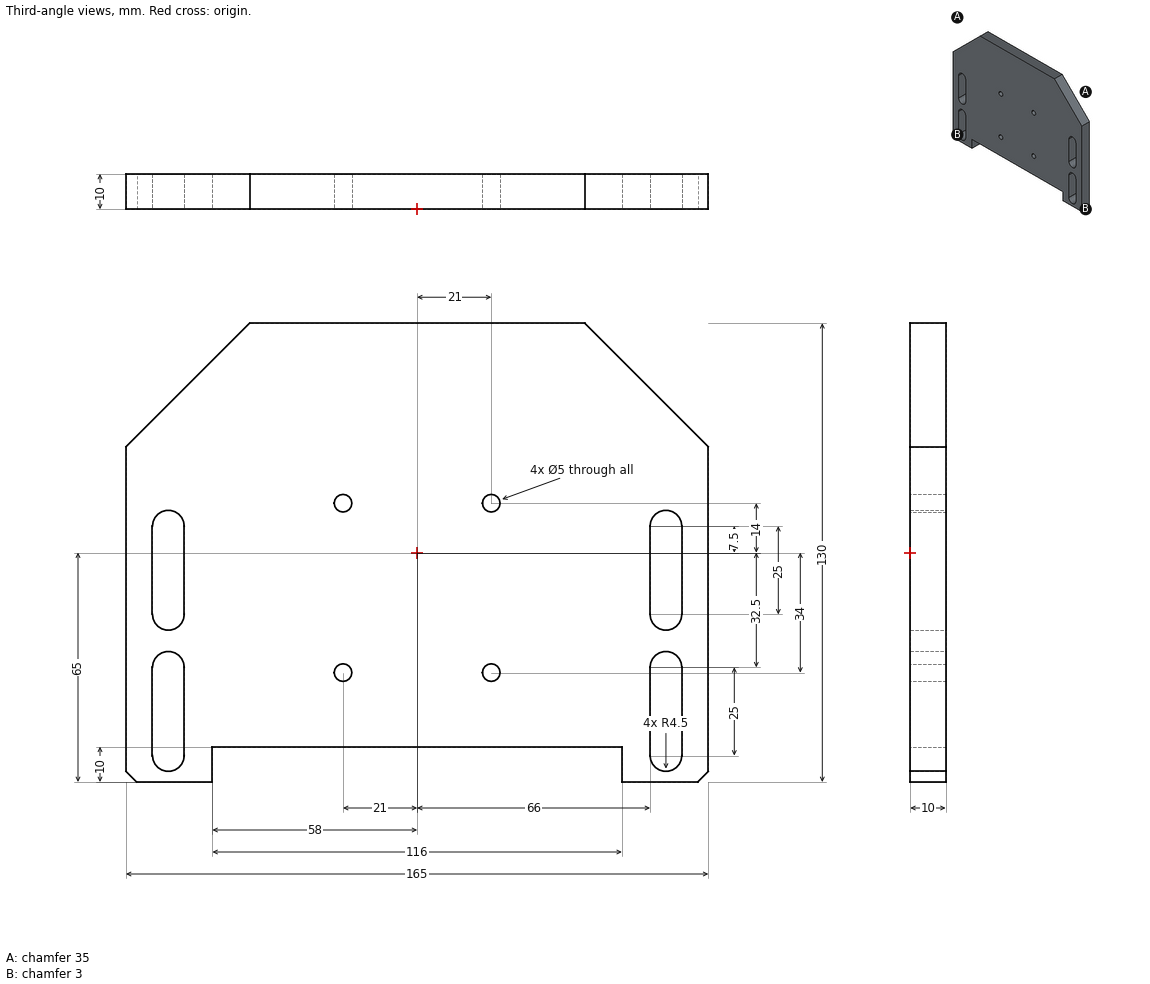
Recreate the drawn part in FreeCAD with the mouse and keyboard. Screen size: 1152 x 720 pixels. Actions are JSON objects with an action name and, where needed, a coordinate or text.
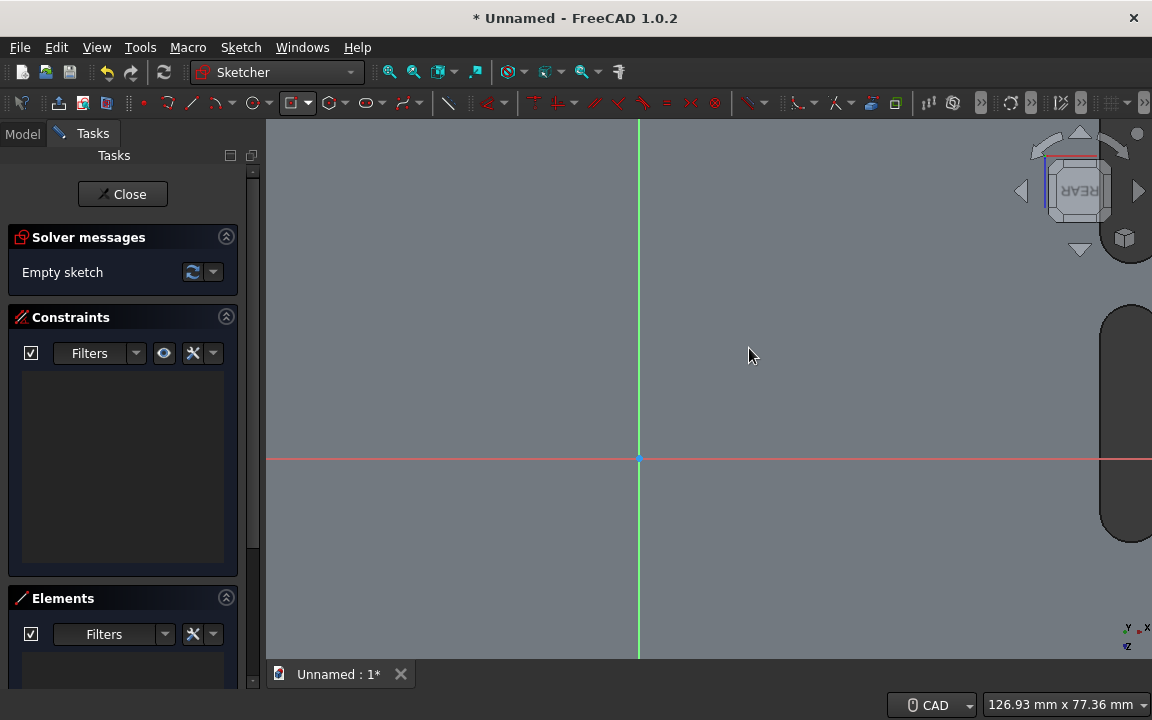
{"action": "left_click", "coordinate": [254, 104]}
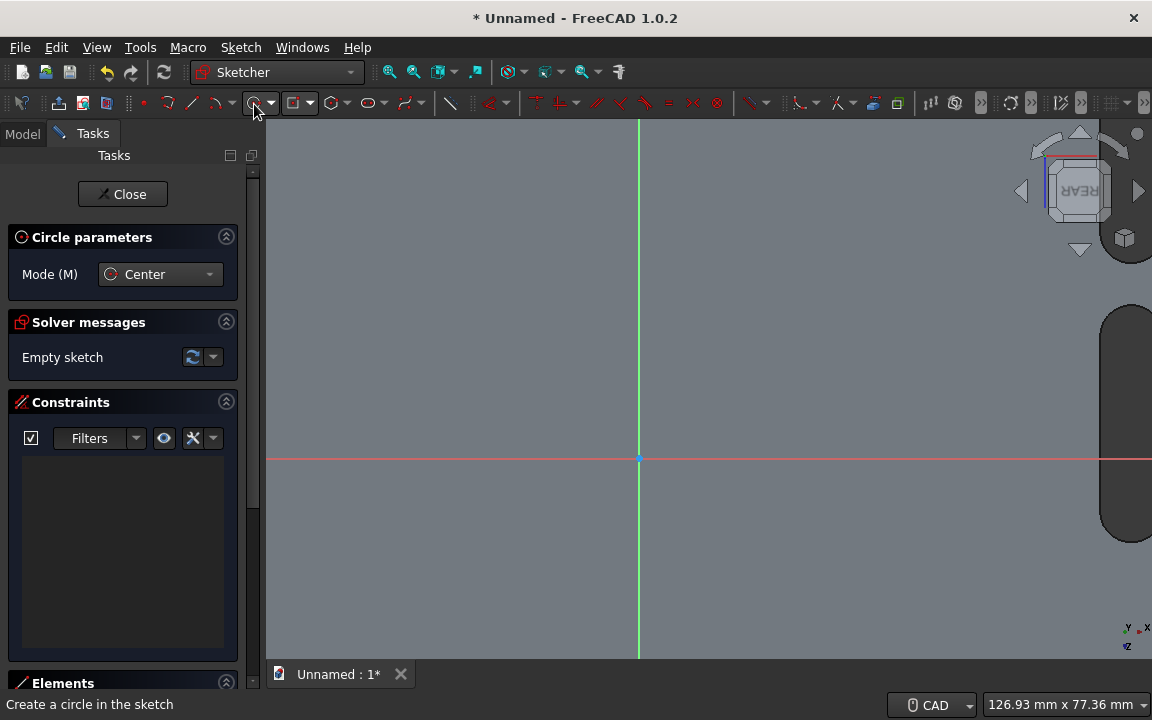
{"action": "scroll", "coordinate": [786, 556], "scroll_direction": "up", "scroll_amount": 2}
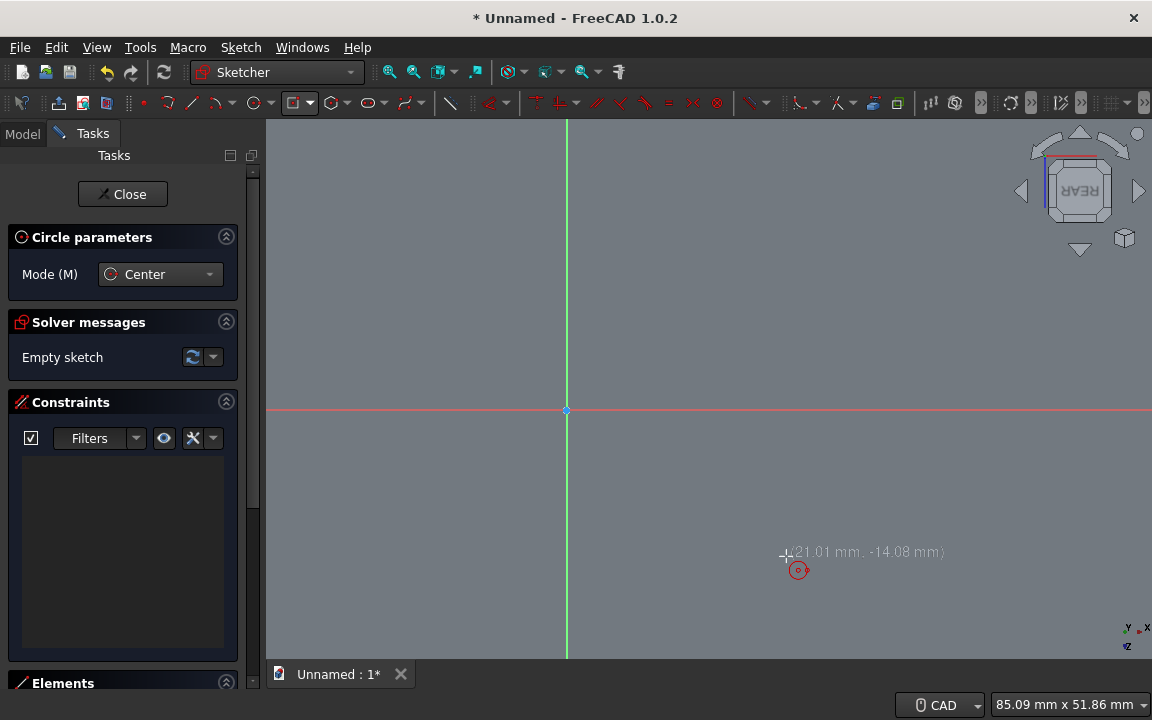
{"action": "left_click", "coordinate": [786, 556]}
{"action": "left_click", "coordinate": [804, 538]}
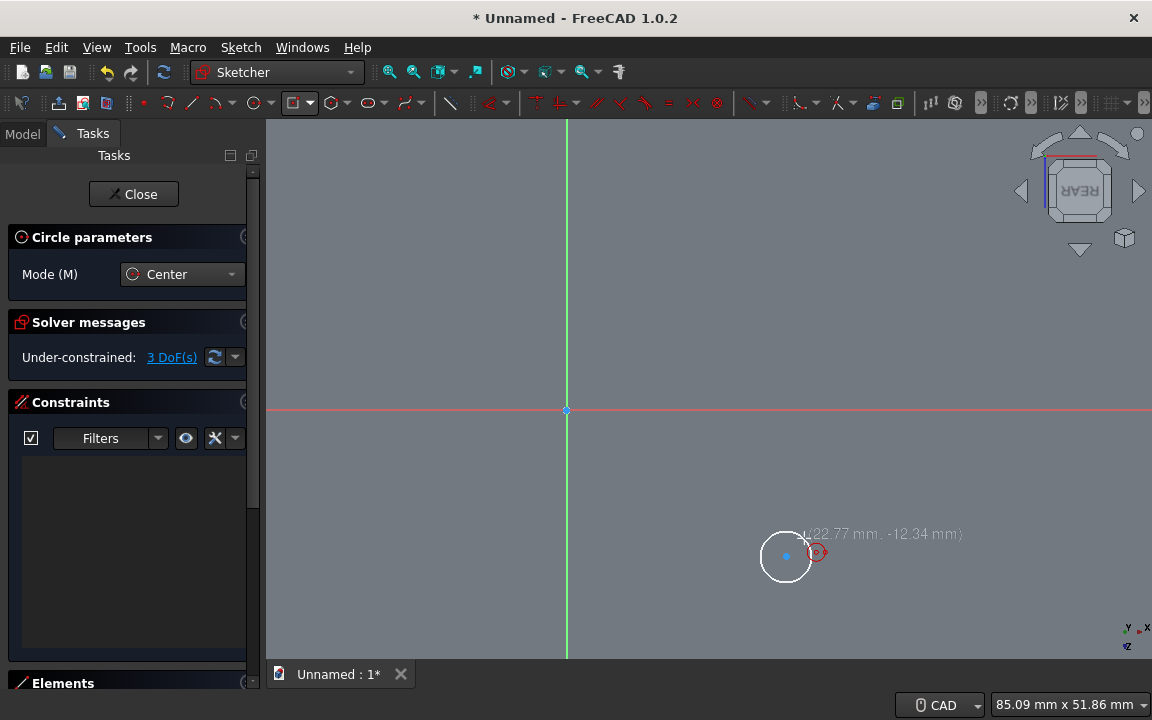
{"action": "scroll", "coordinate": [790, 557], "scroll_direction": "down", "scroll_amount": 2}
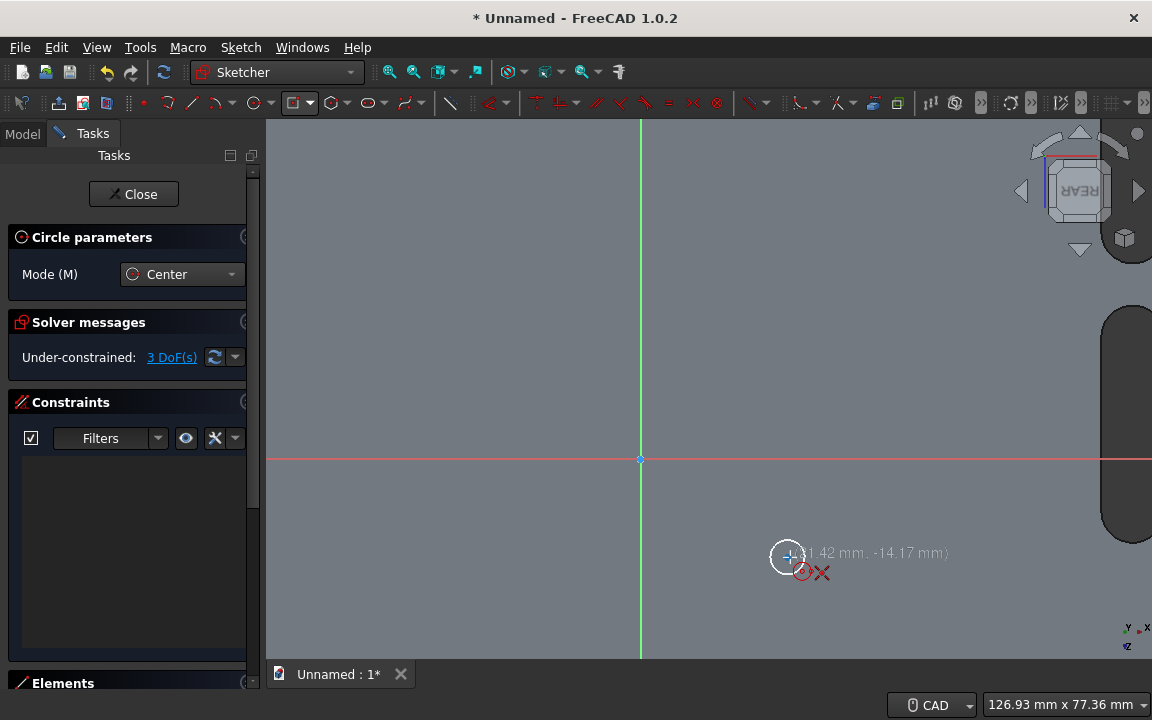
{"action": "scroll", "coordinate": [787, 222], "scroll_direction": "up", "scroll_amount": 2}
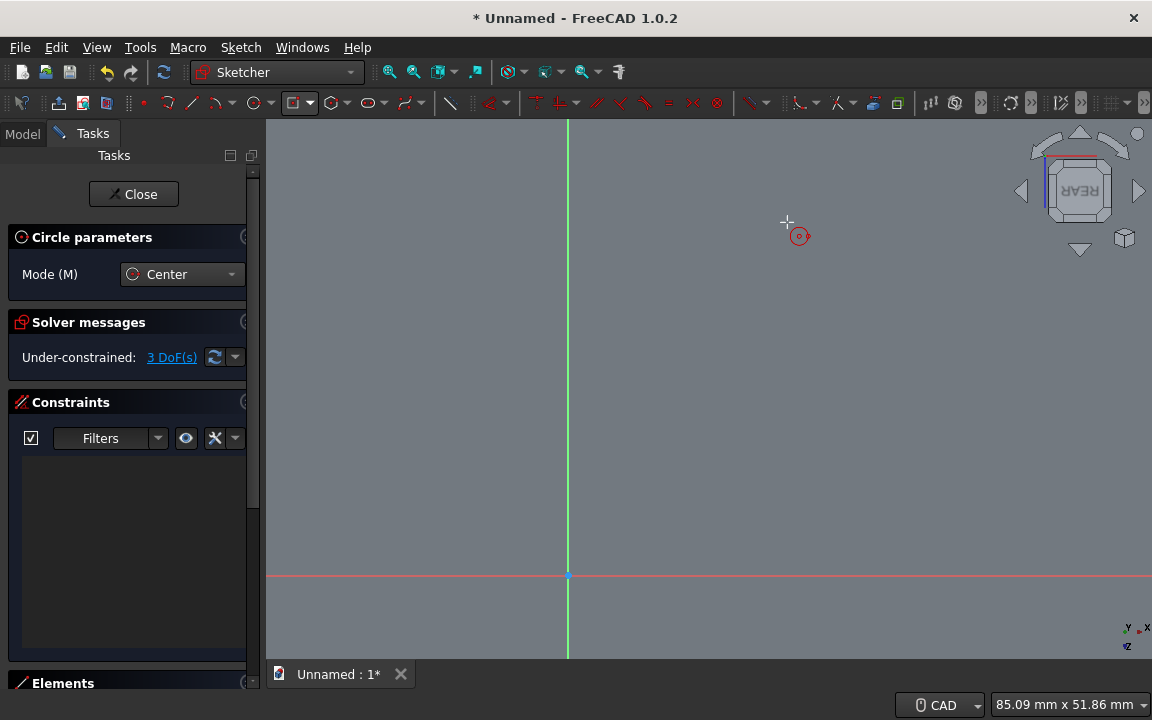
{"action": "left_click", "coordinate": [787, 222]}
{"action": "left_click", "coordinate": [805, 203]}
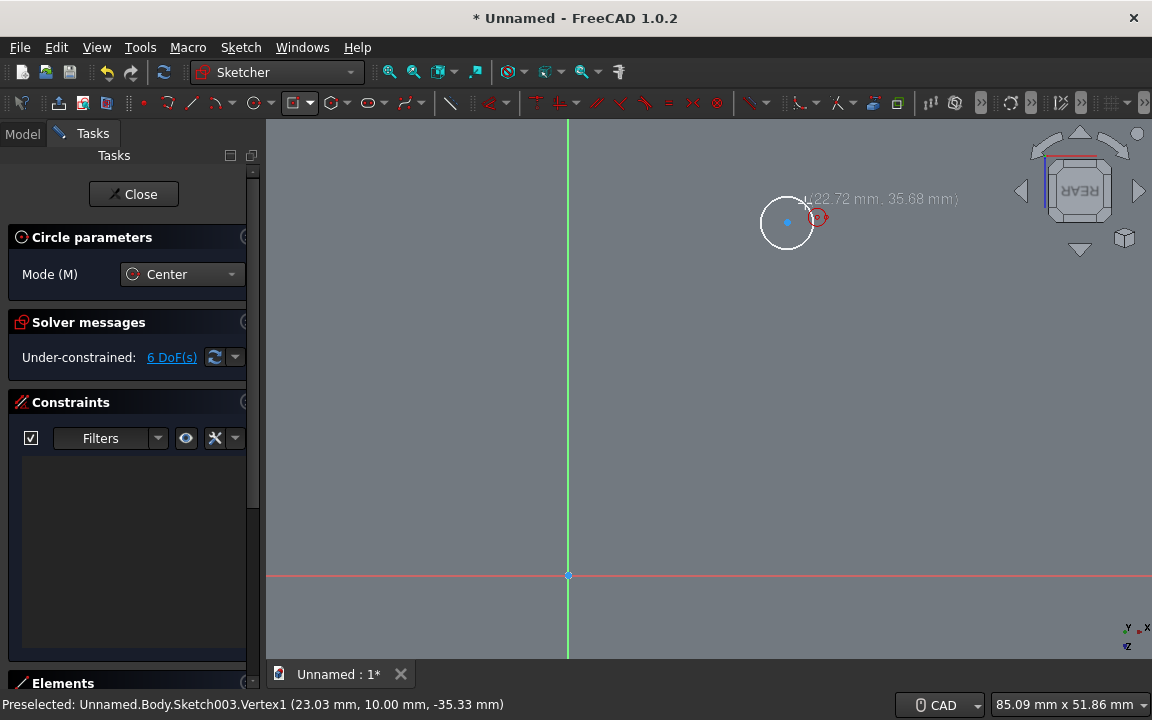
{"action": "left_click", "coordinate": [350, 222]}
{"action": "left_click", "coordinate": [368, 203]}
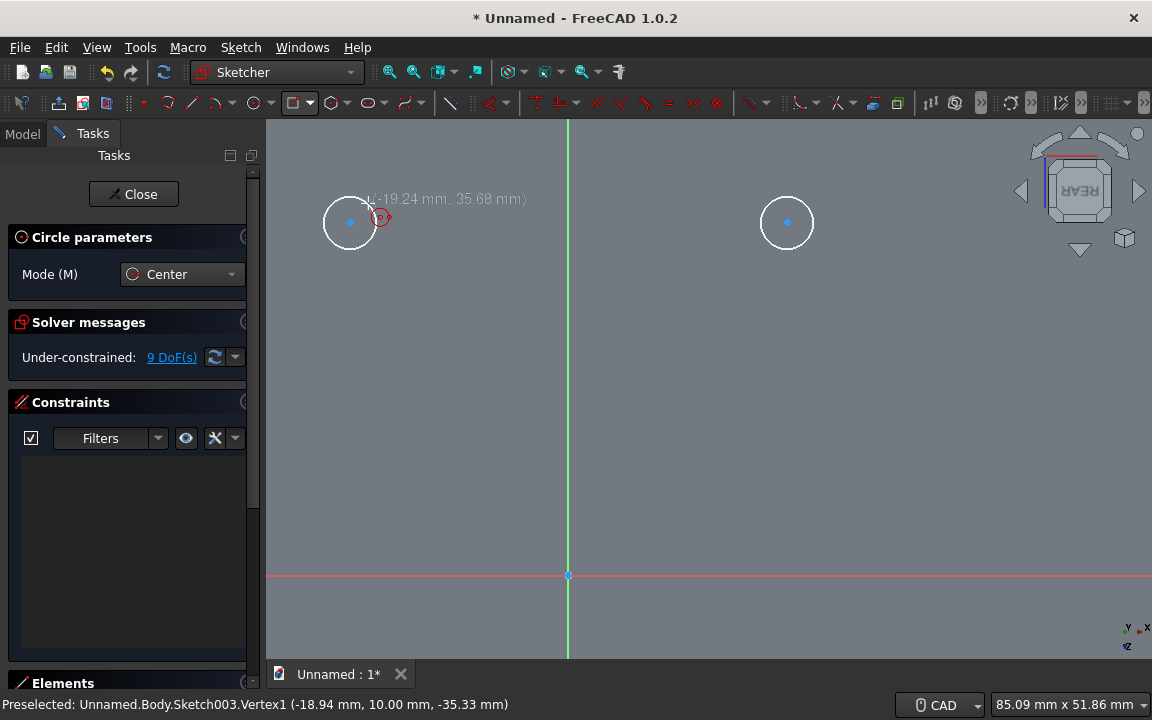
{"action": "scroll", "coordinate": [787, 221], "scroll_direction": "down", "scroll_amount": 2}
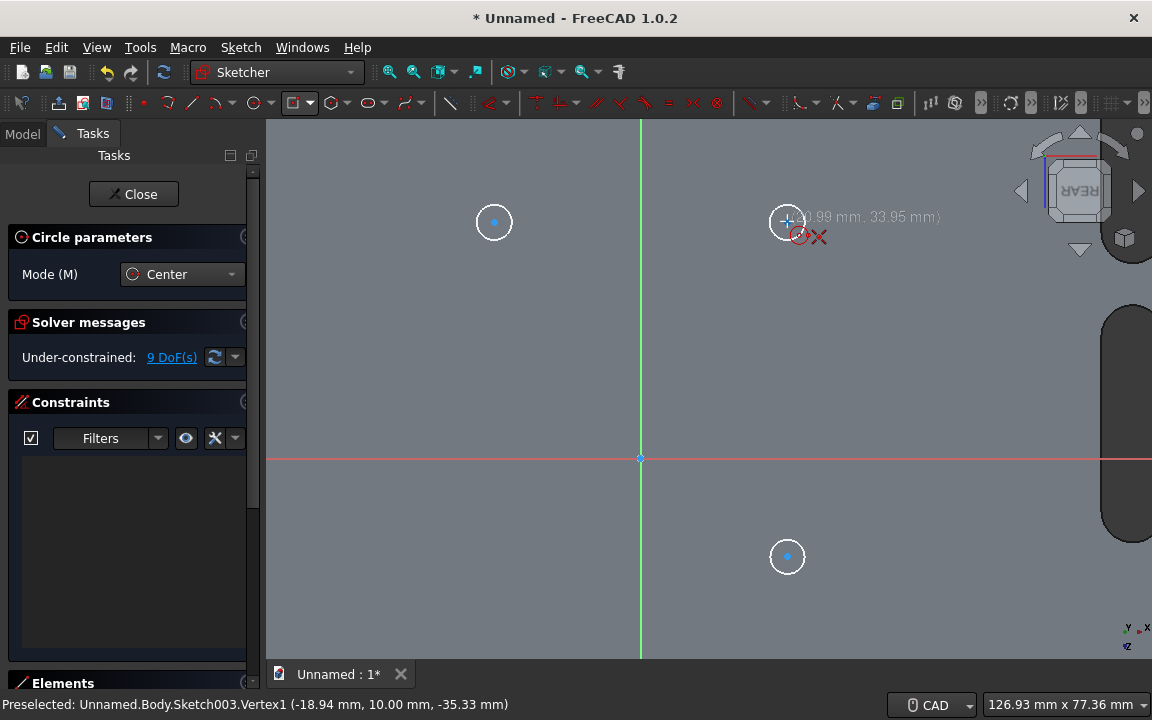
{"action": "scroll", "coordinate": [494, 556], "scroll_direction": "up", "scroll_amount": 2}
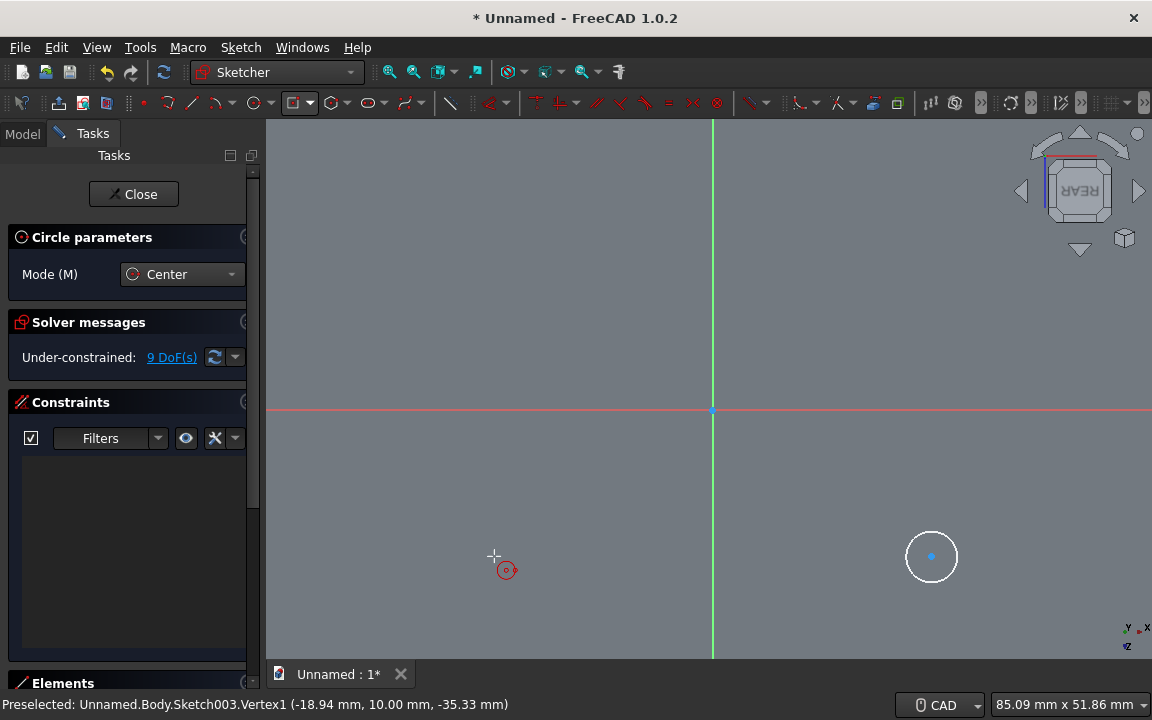
{"action": "left_click", "coordinate": [494, 556]}
{"action": "left_click", "coordinate": [512, 538]}
{"action": "key", "text": "Escape"}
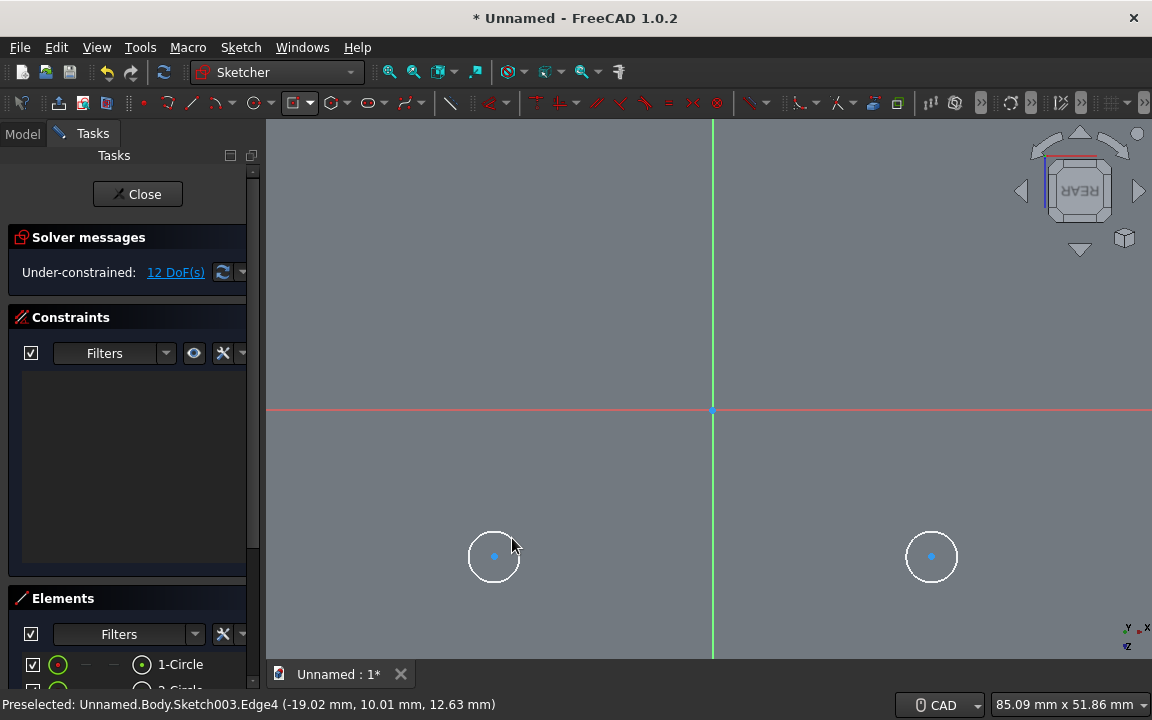
{"action": "left_click", "coordinate": [950, 539]}